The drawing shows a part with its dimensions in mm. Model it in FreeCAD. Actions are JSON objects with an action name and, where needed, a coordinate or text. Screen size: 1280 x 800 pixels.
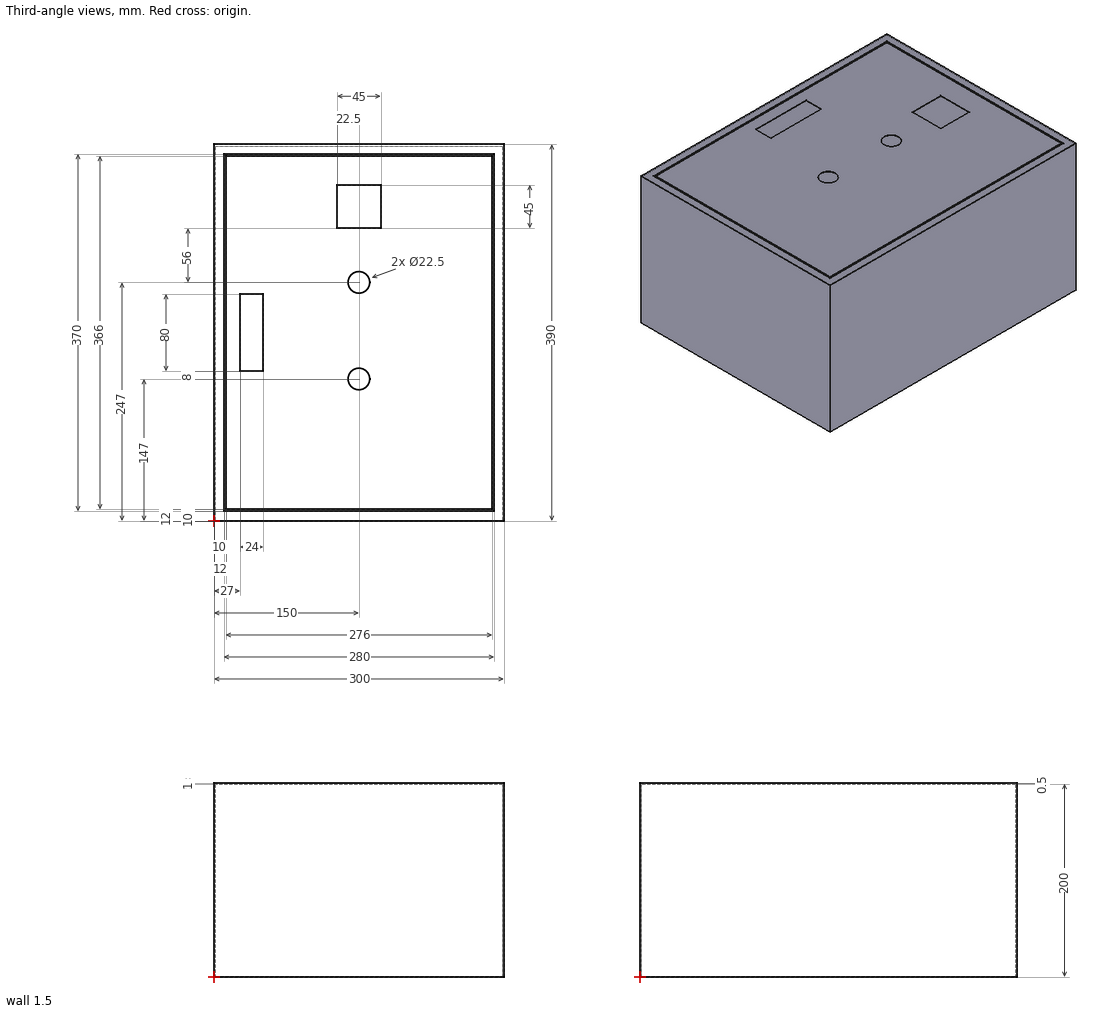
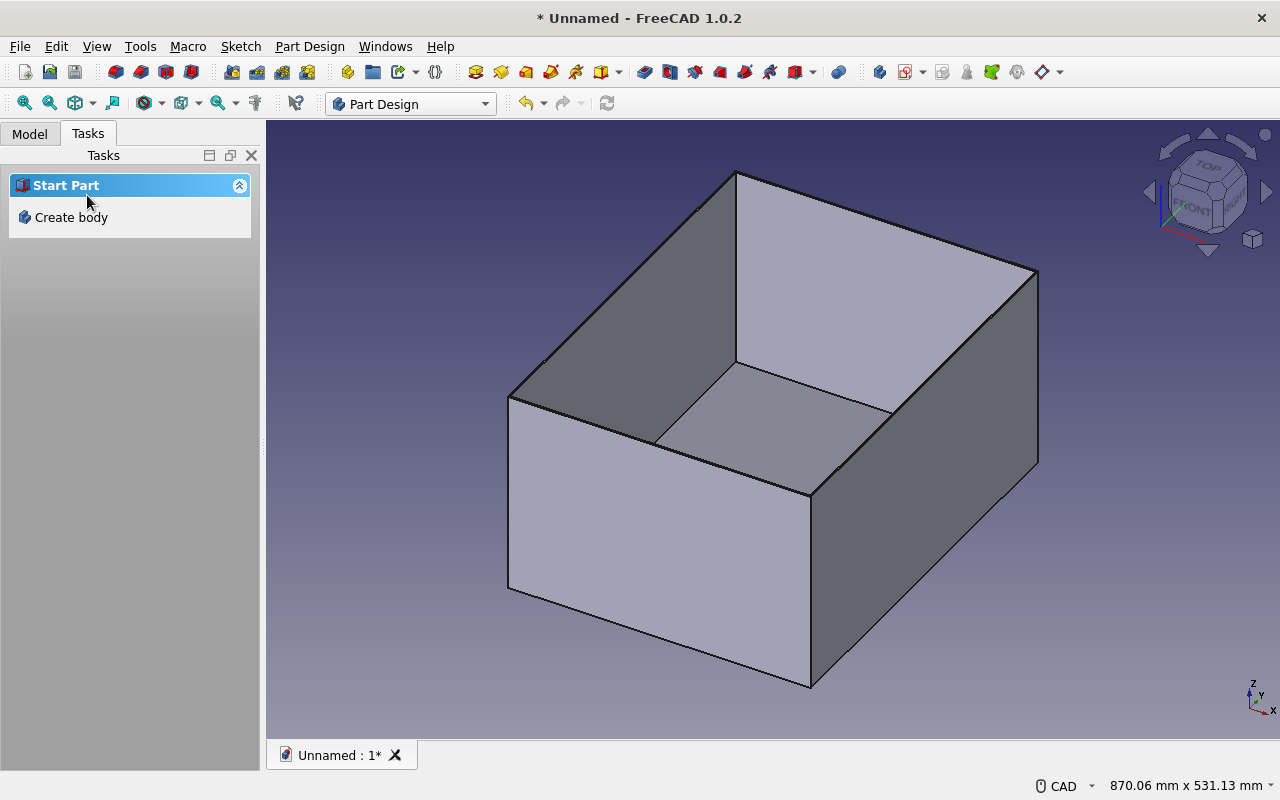
{"action": "scroll", "coordinate": [961, 346], "scroll_direction": "up", "scroll_amount": 15}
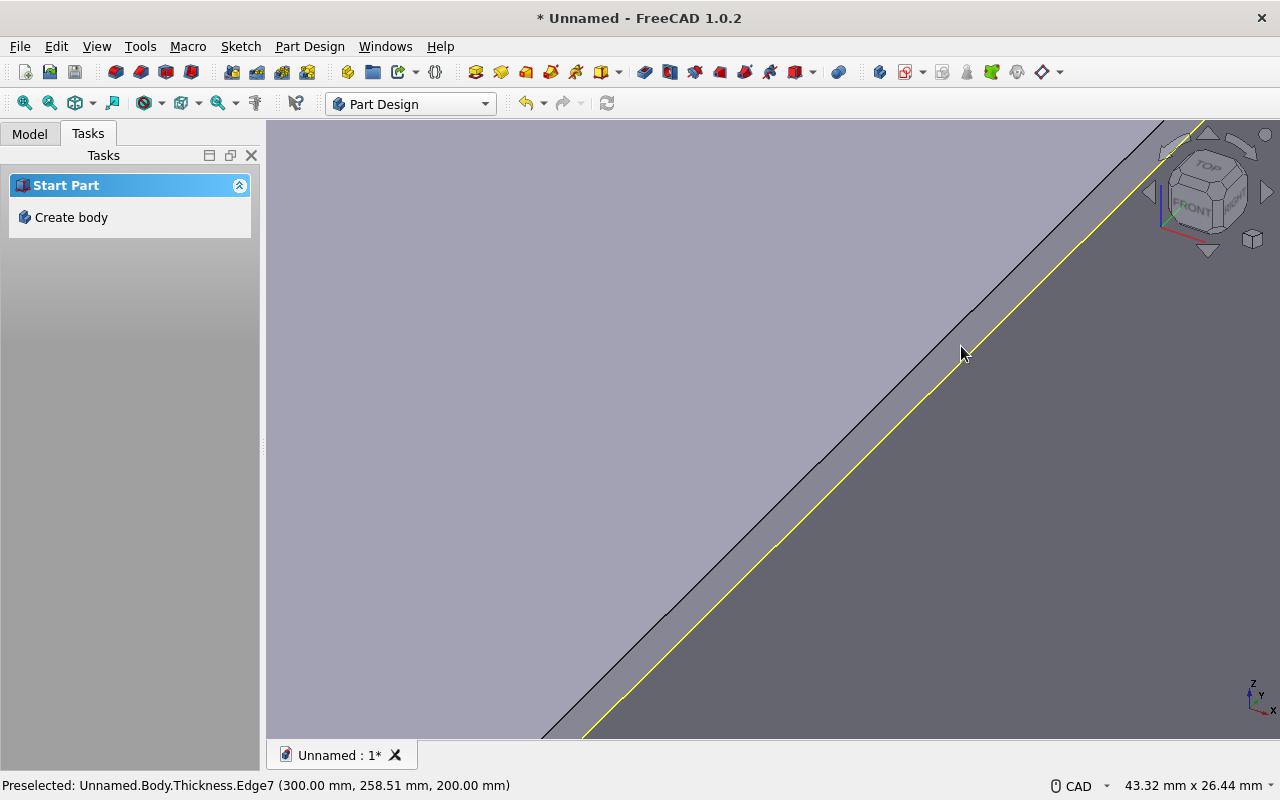
{"action": "left_click", "coordinate": [957, 351]}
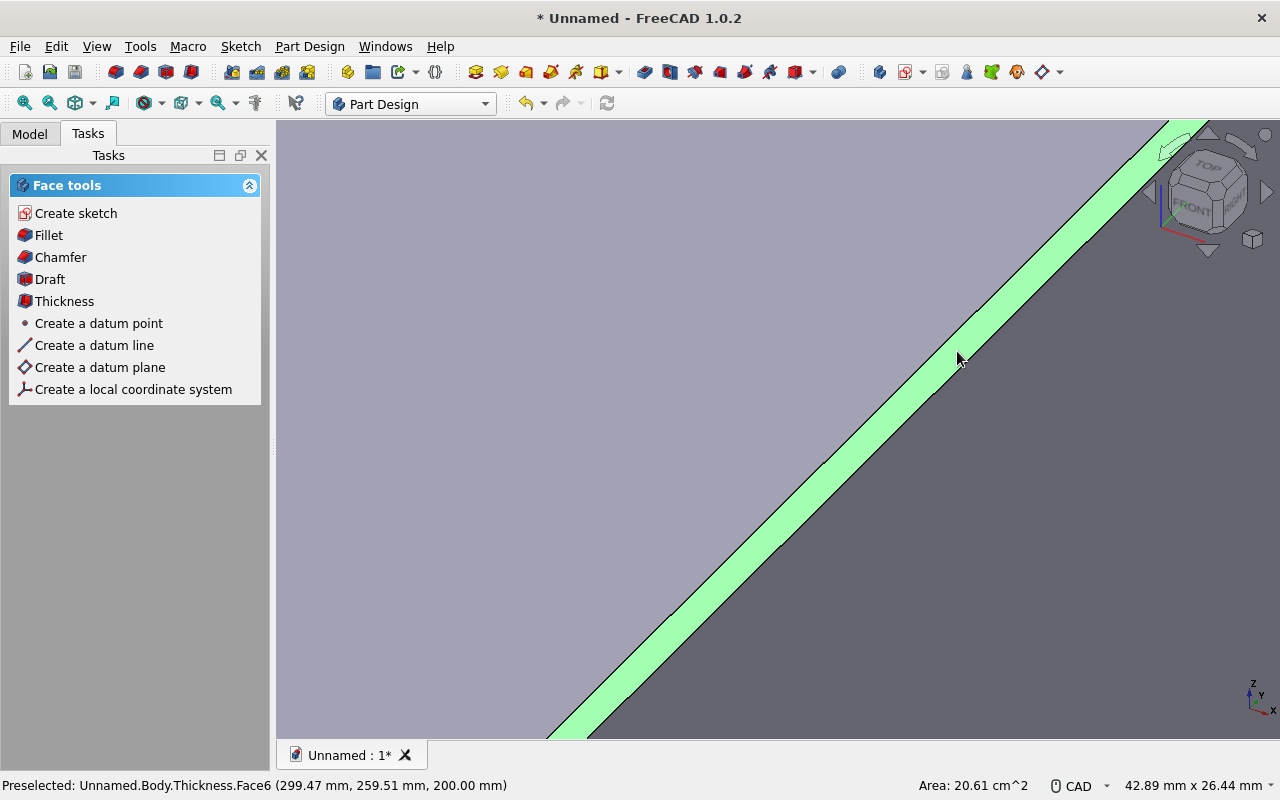
{"action": "left_click", "coordinate": [904, 72]}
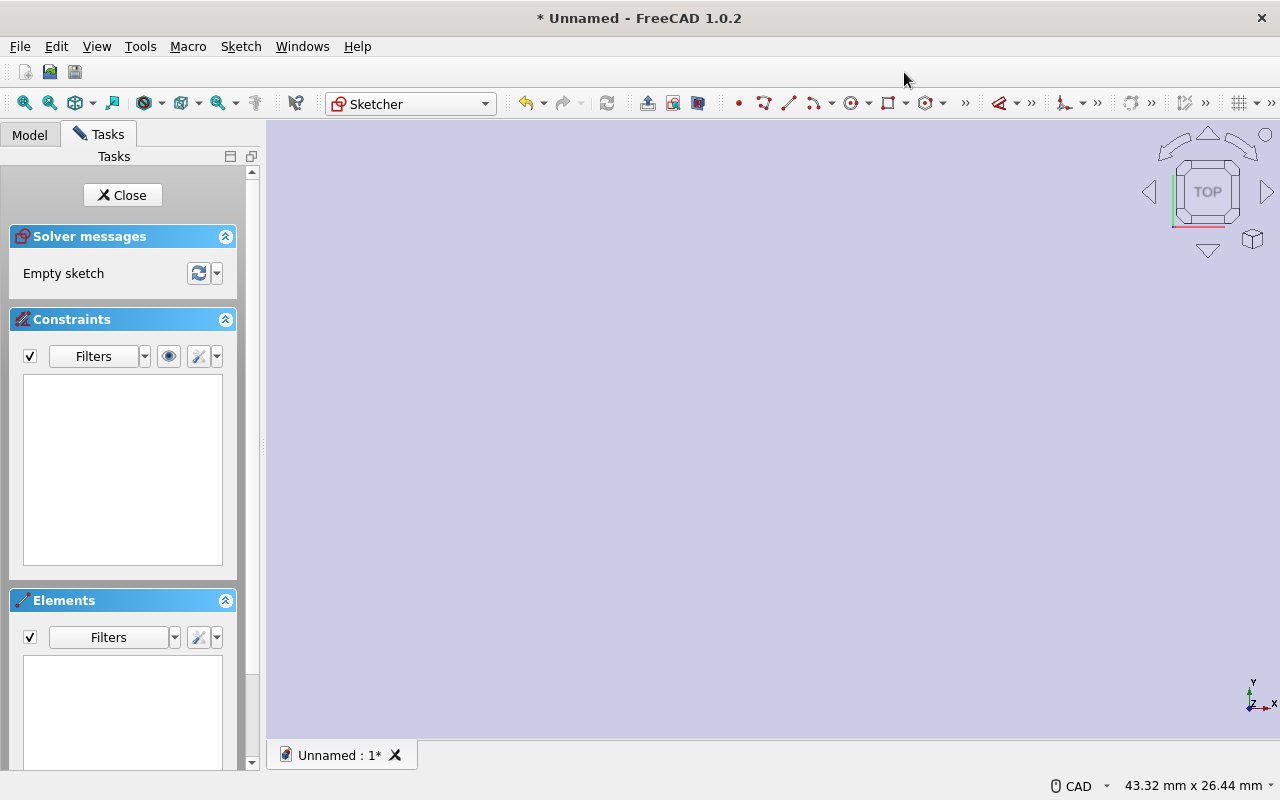
{"action": "scroll", "coordinate": [840, 294], "scroll_direction": "down", "scroll_amount": 15}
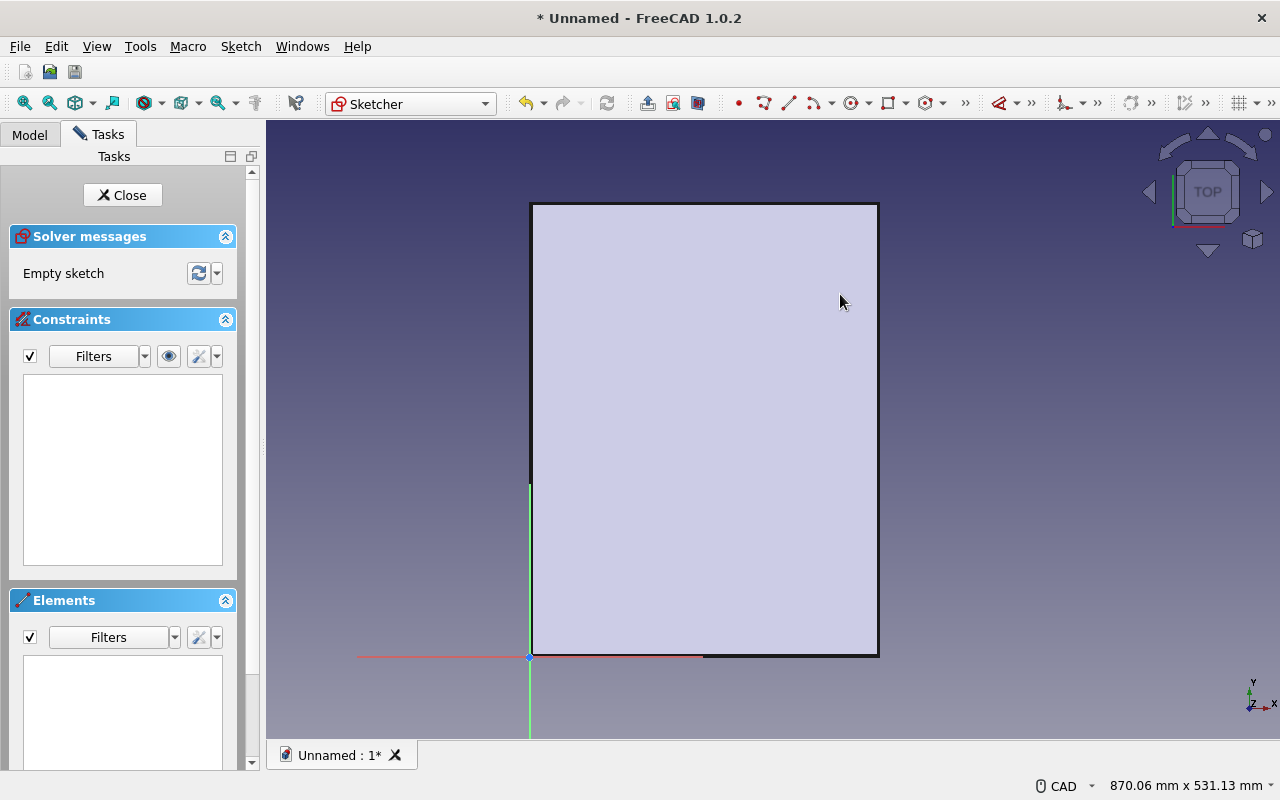
{"action": "left_click", "coordinate": [888, 104]}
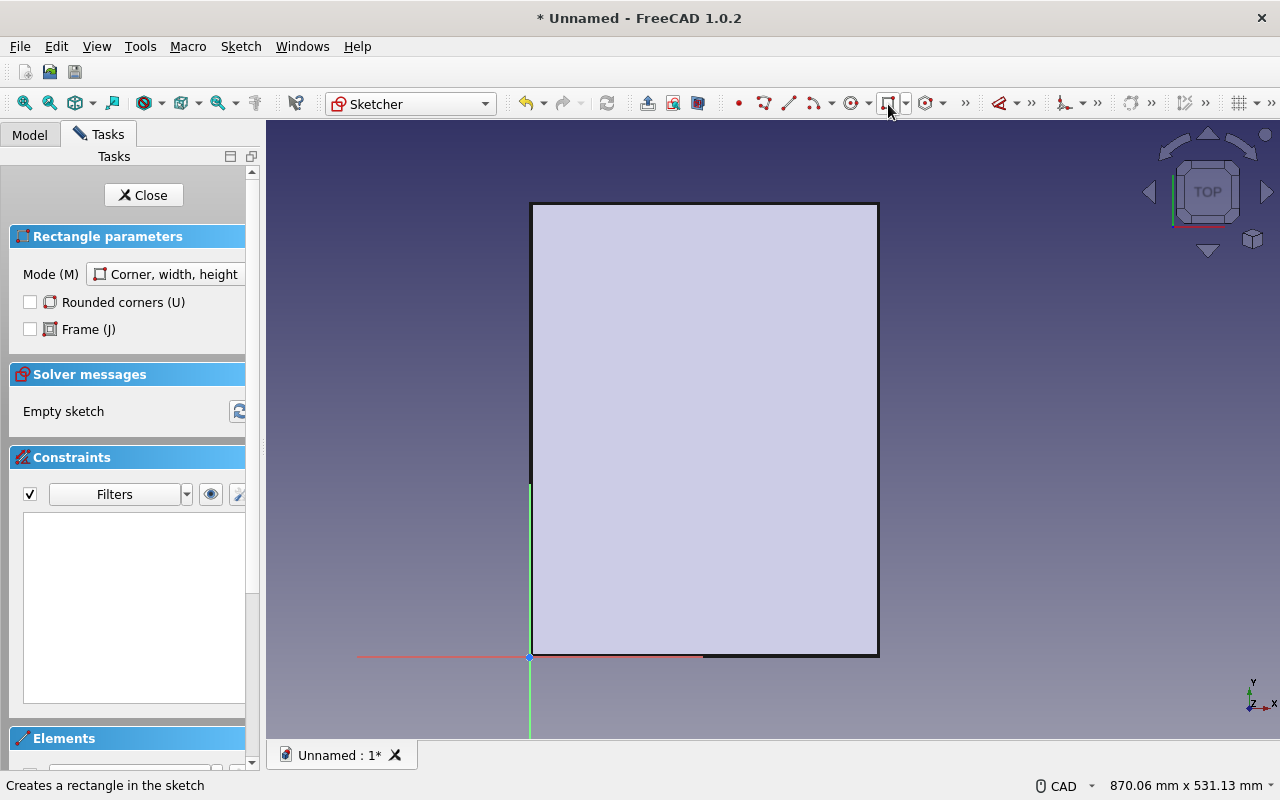
{"action": "left_click", "coordinate": [530, 657]}
{"action": "mouse_move", "coordinate": [879, 203]}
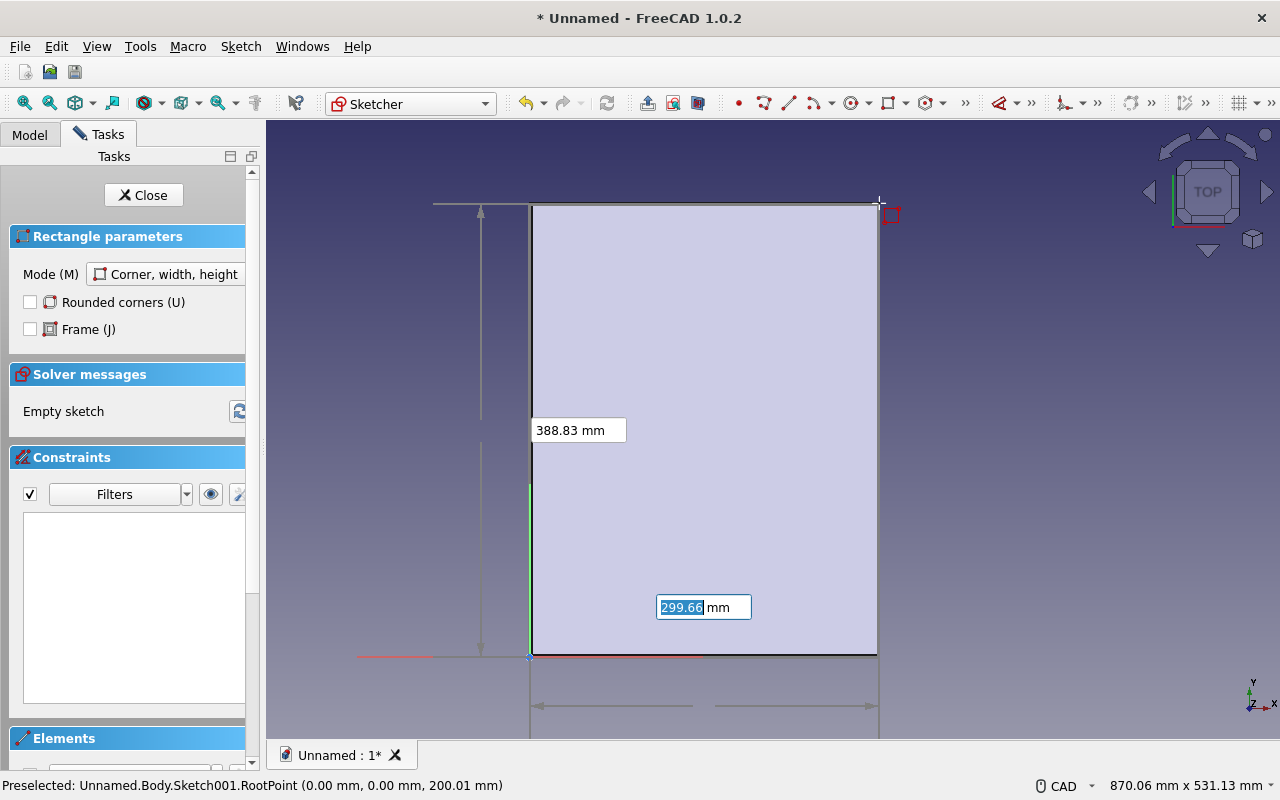
{"action": "type", "text": "300"}
{"action": "key", "text": "Tab"}
{"action": "type", "text": "390"}
{"action": "key", "text": "Return"}
{"action": "key", "text": "Escape"}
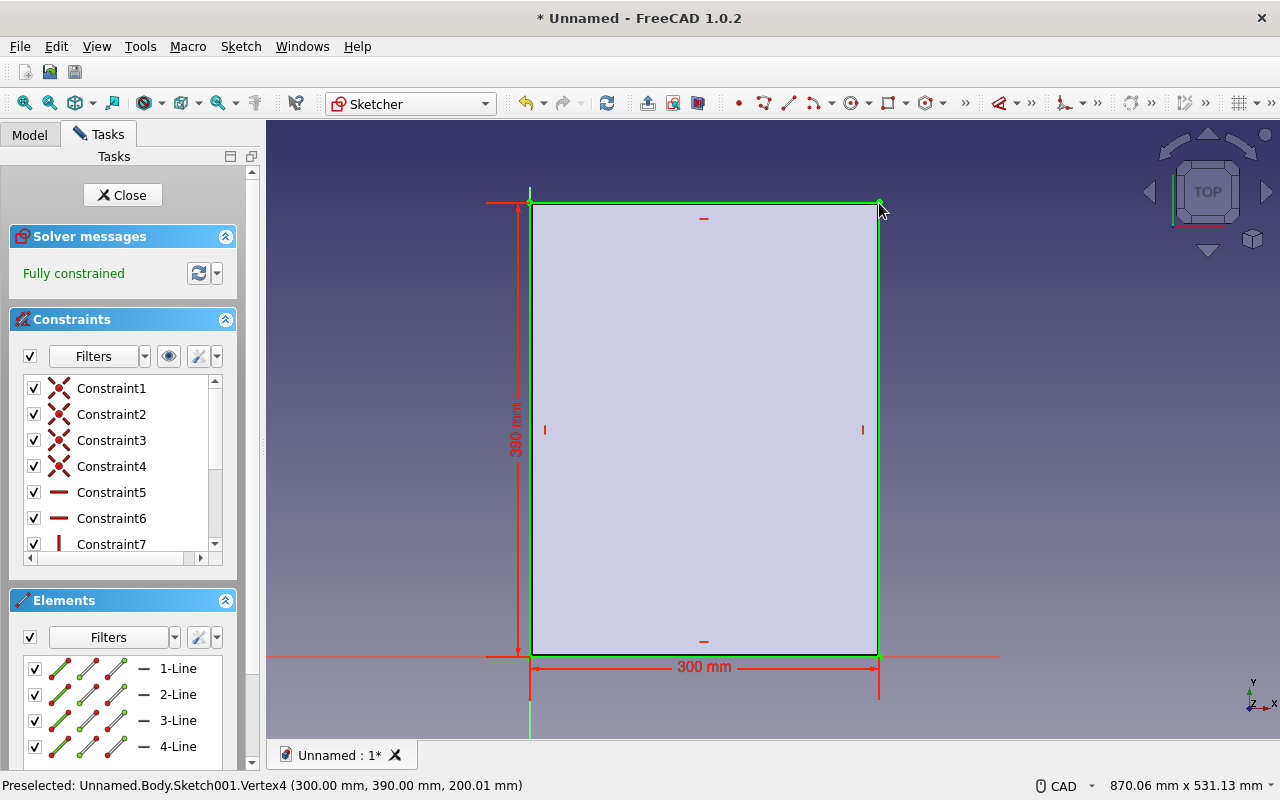
{"action": "left_click", "coordinate": [123, 195]}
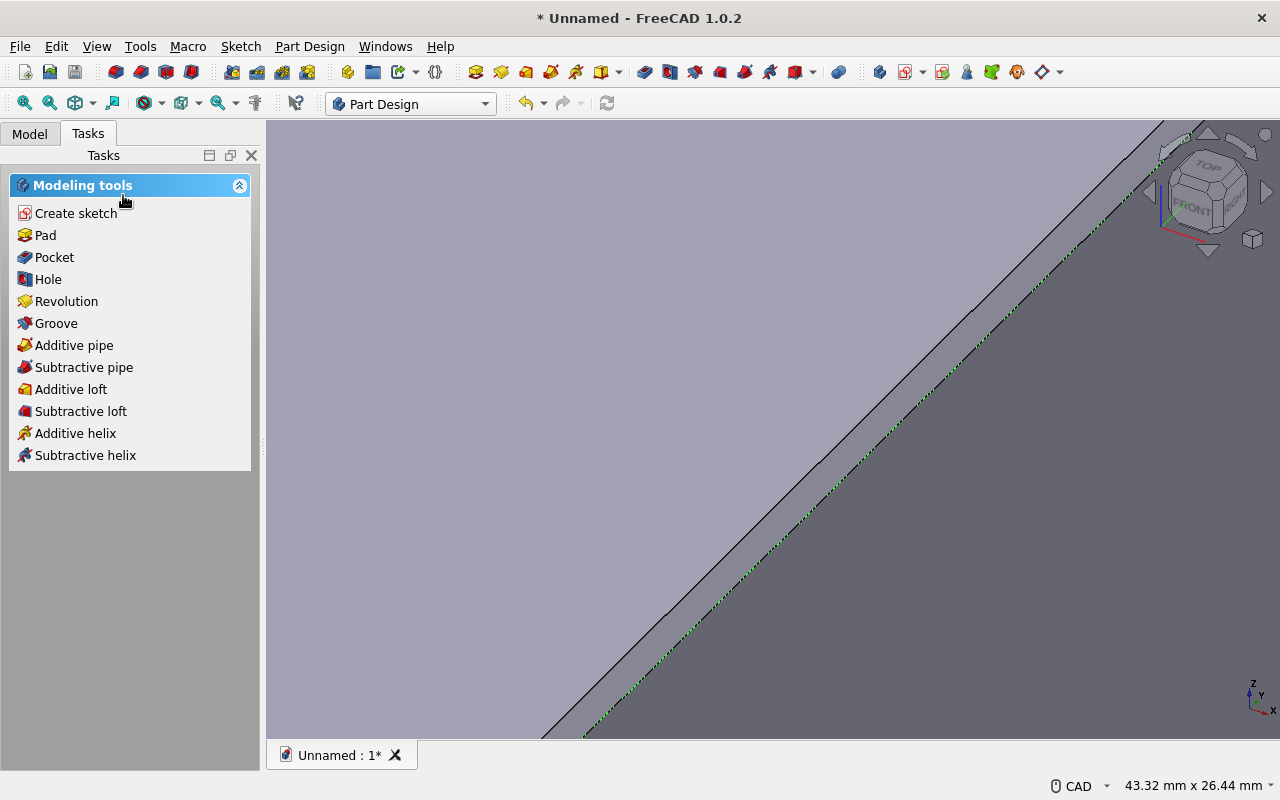
{"action": "left_click", "coordinate": [476, 72]}